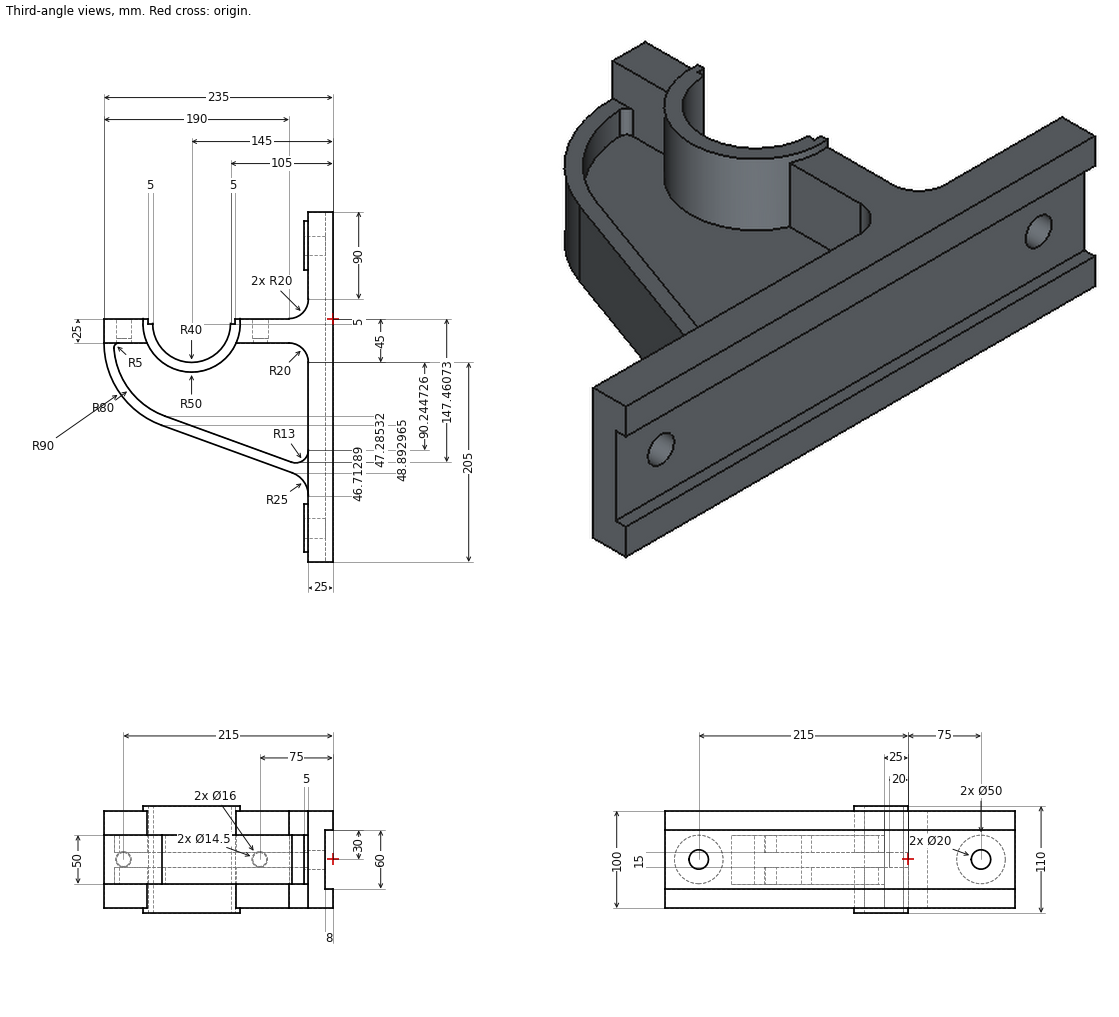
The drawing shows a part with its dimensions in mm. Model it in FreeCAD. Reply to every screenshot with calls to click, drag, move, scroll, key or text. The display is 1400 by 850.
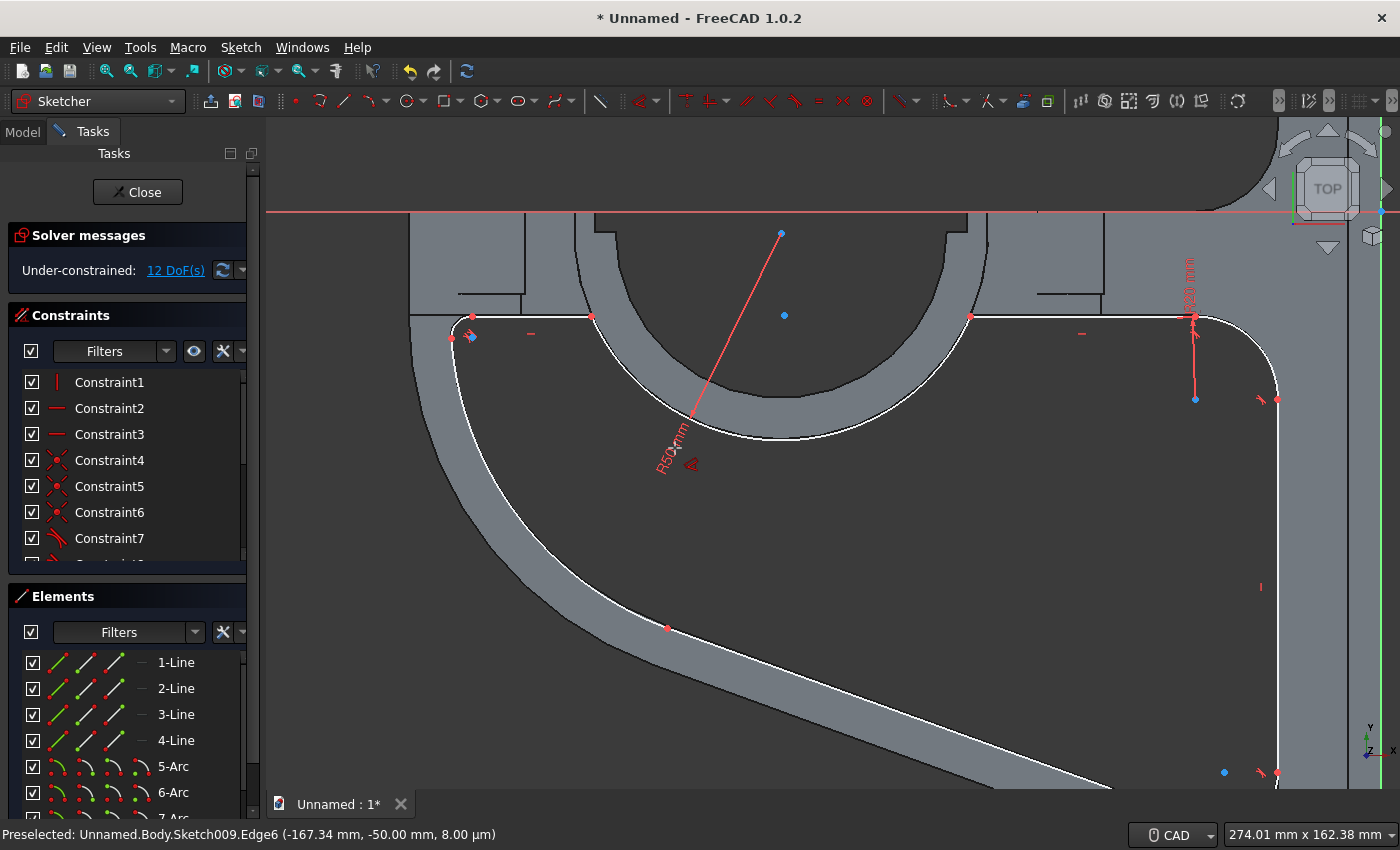
scroll(462, 319, up, 4)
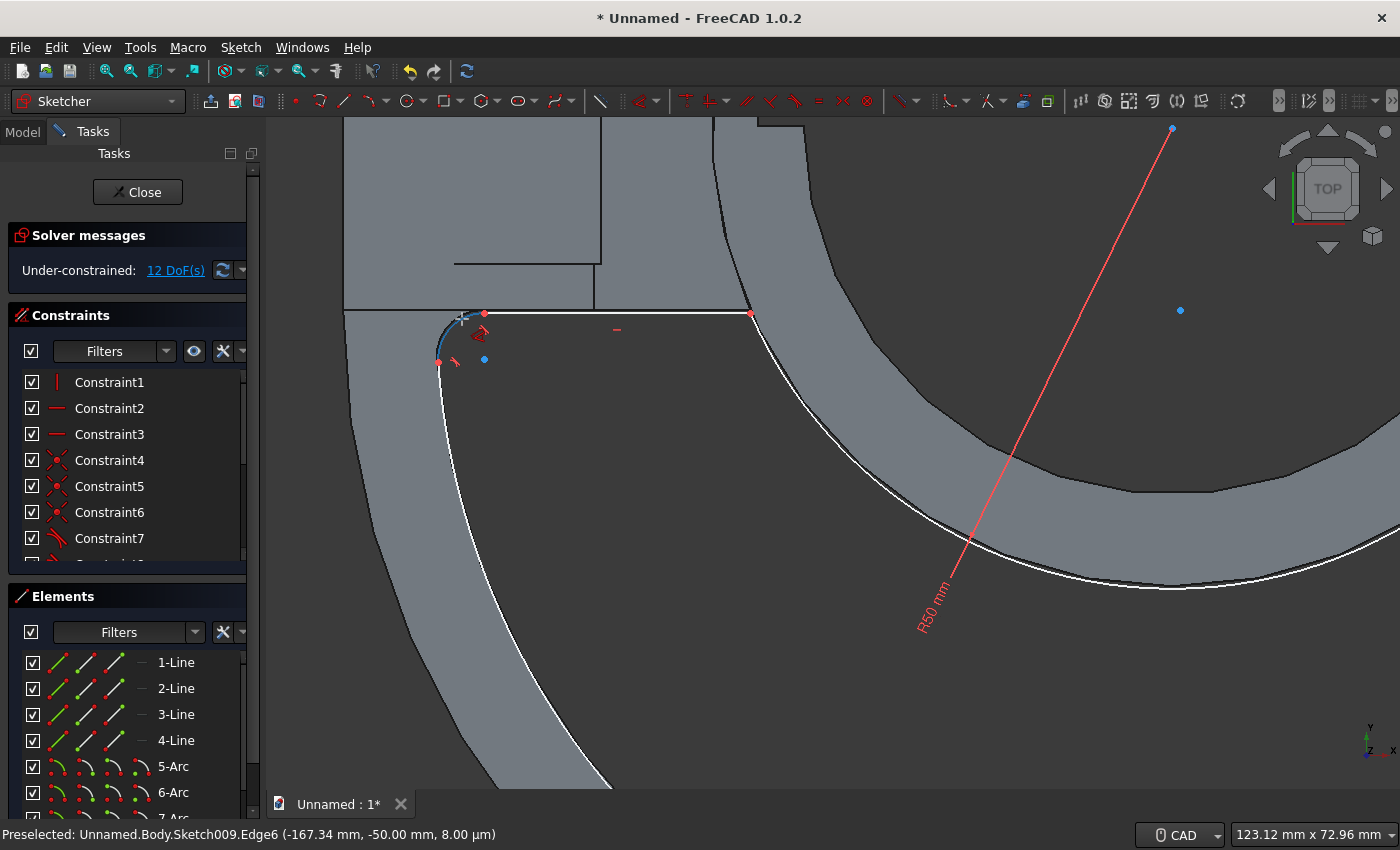
click(463, 319)
click(448, 291)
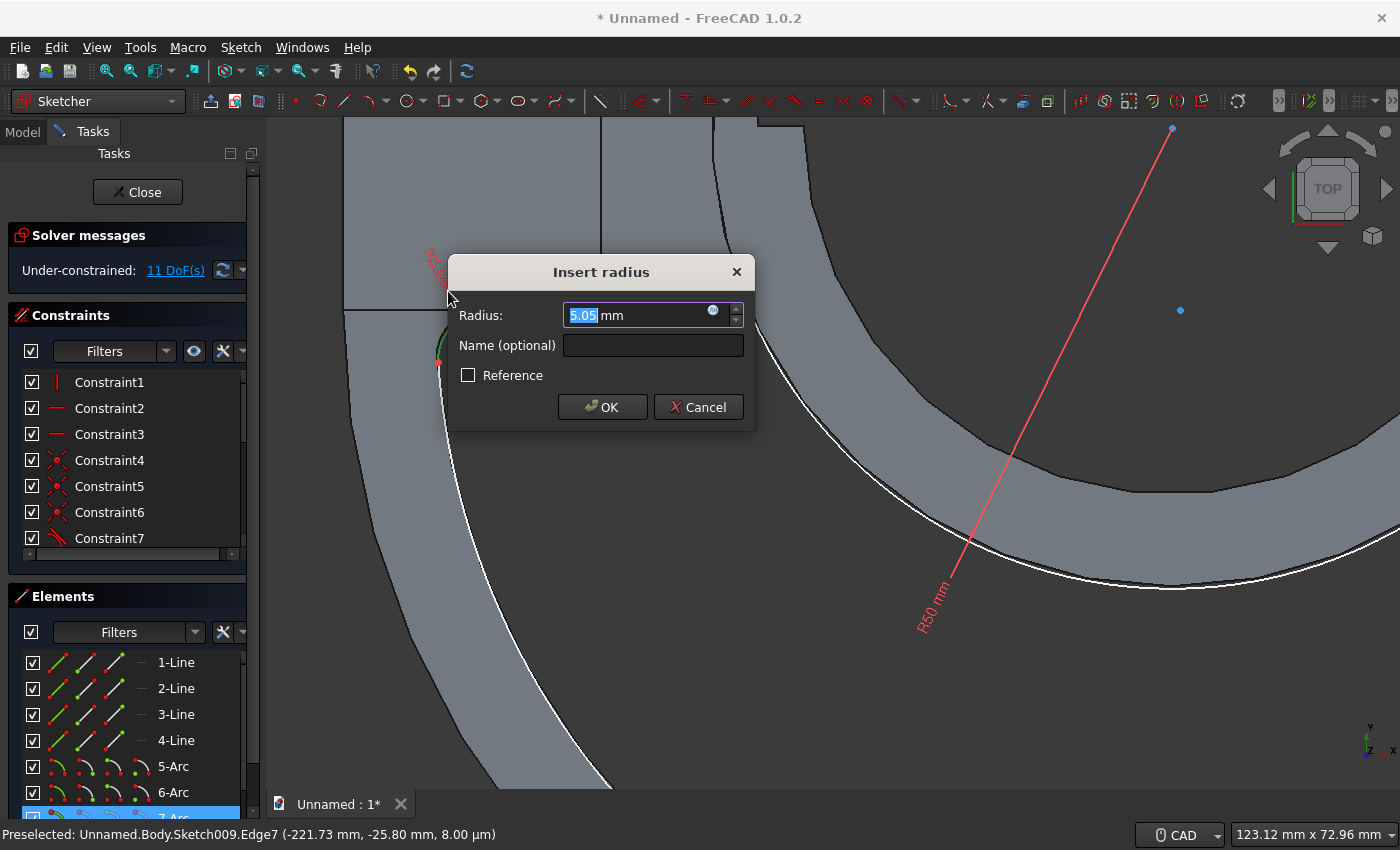
text(5)
key(Return)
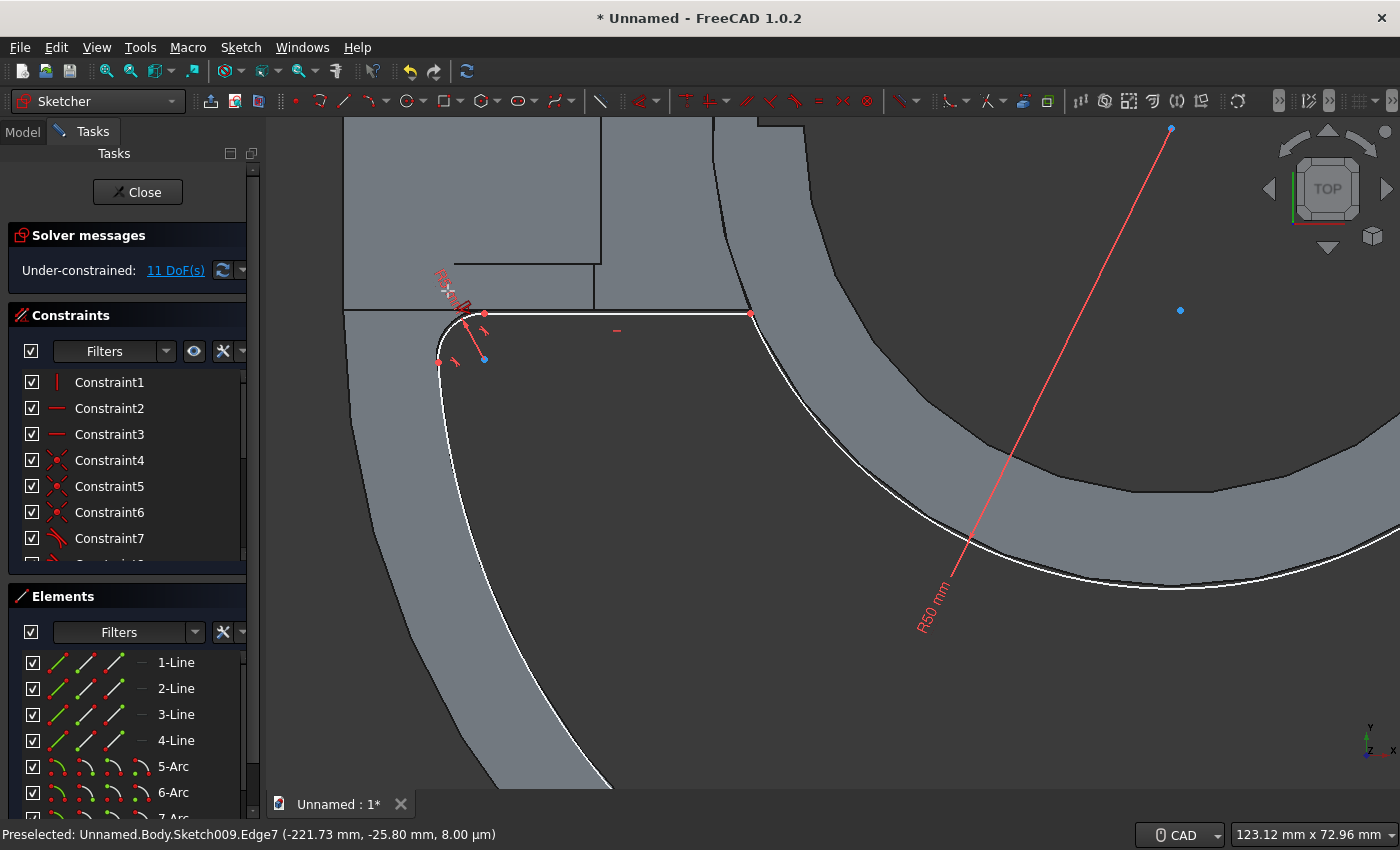
click(499, 609)
click(470, 622)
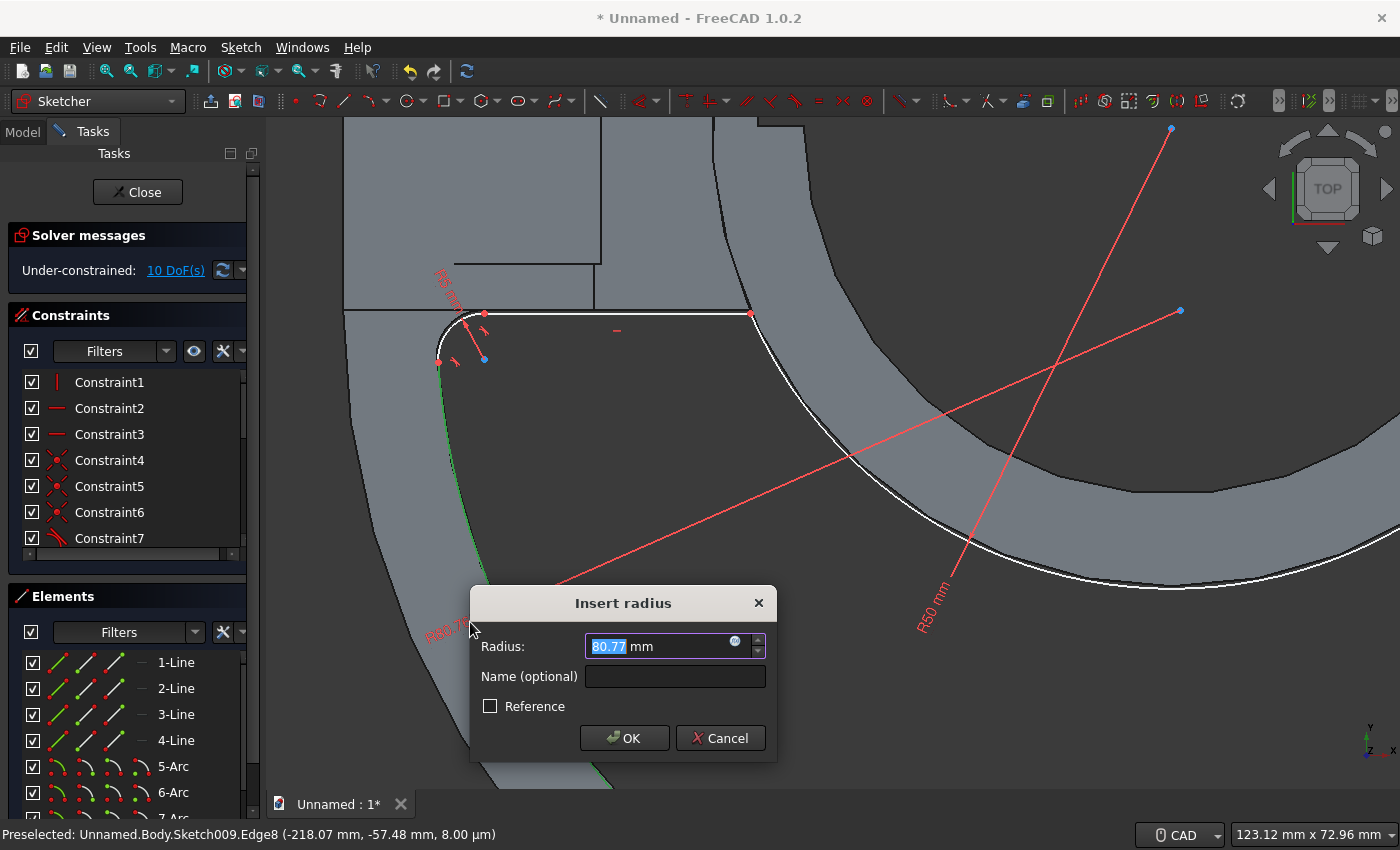
text(80)
key(Return)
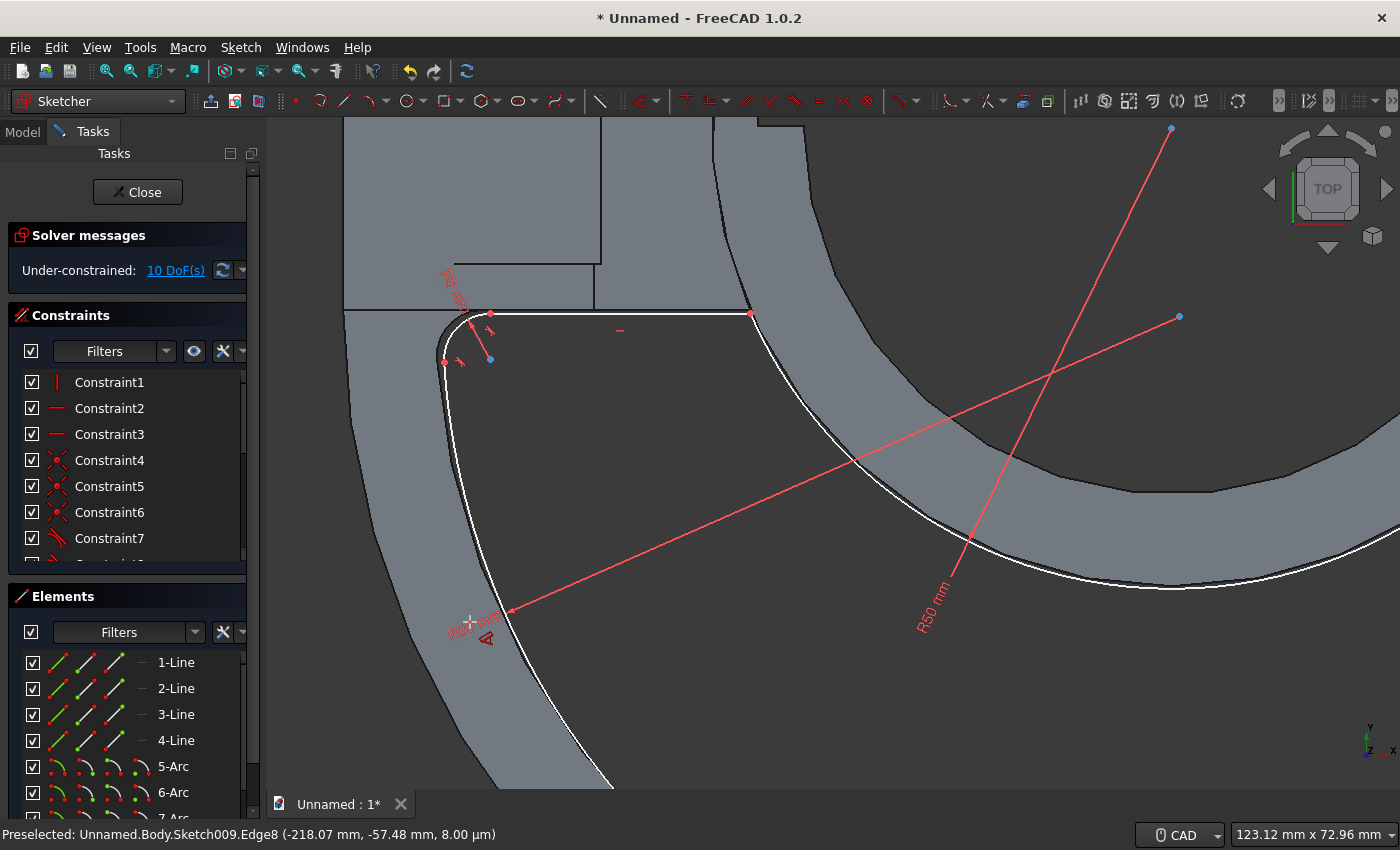
scroll(459, 321, down, 6)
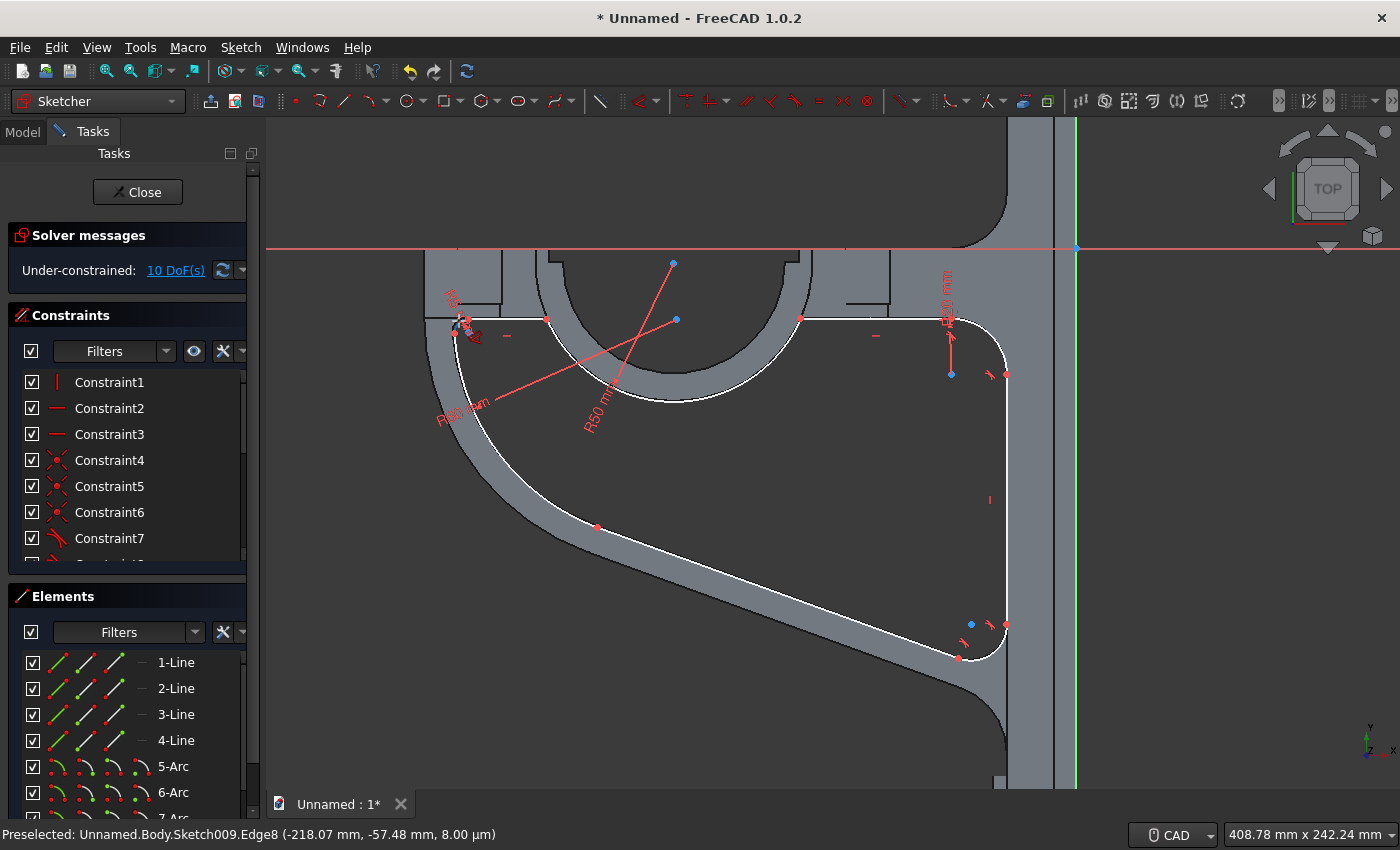
click(979, 660)
click(986, 691)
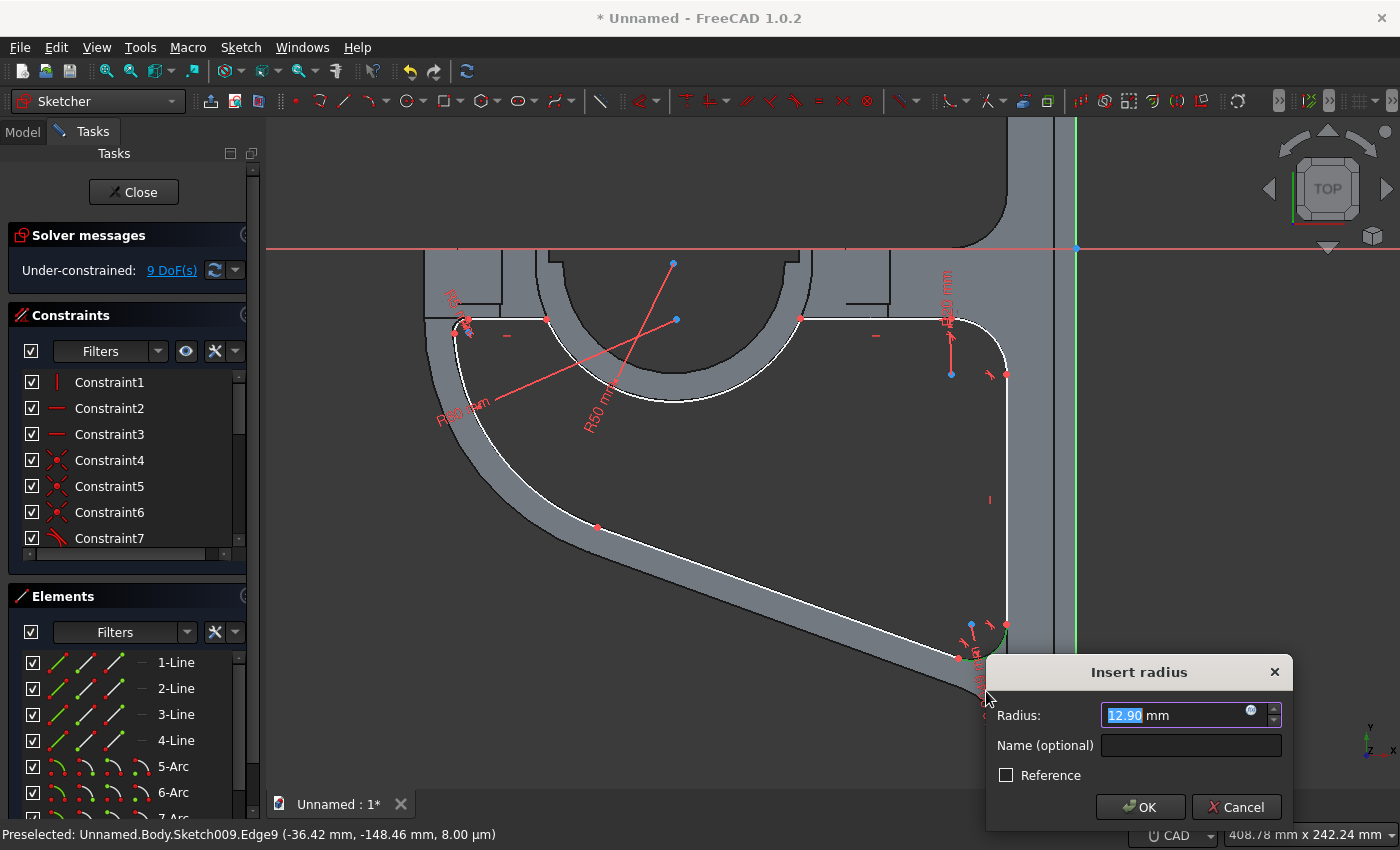
text(13)
key(Return)